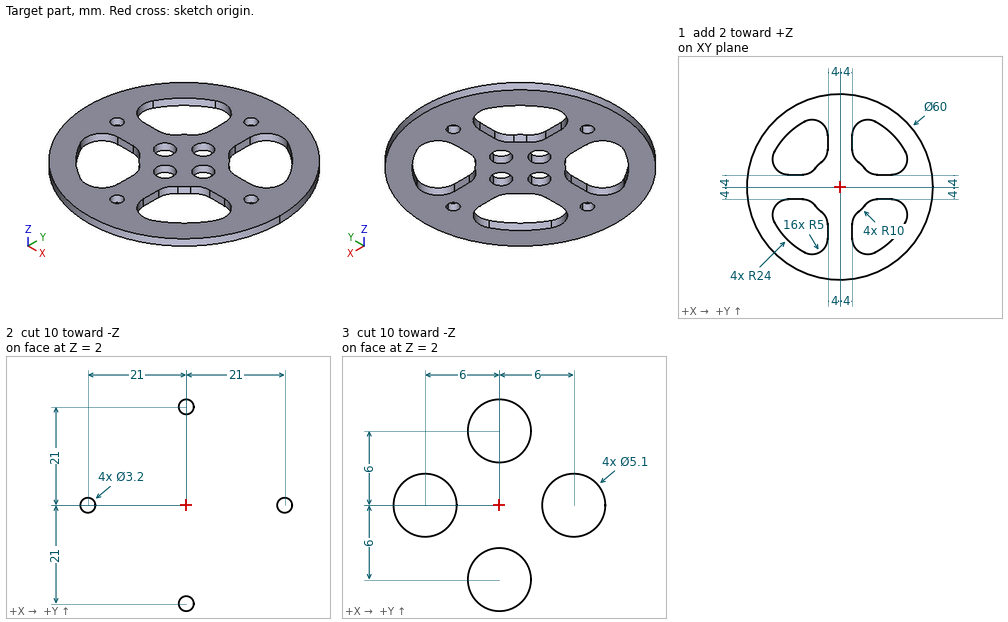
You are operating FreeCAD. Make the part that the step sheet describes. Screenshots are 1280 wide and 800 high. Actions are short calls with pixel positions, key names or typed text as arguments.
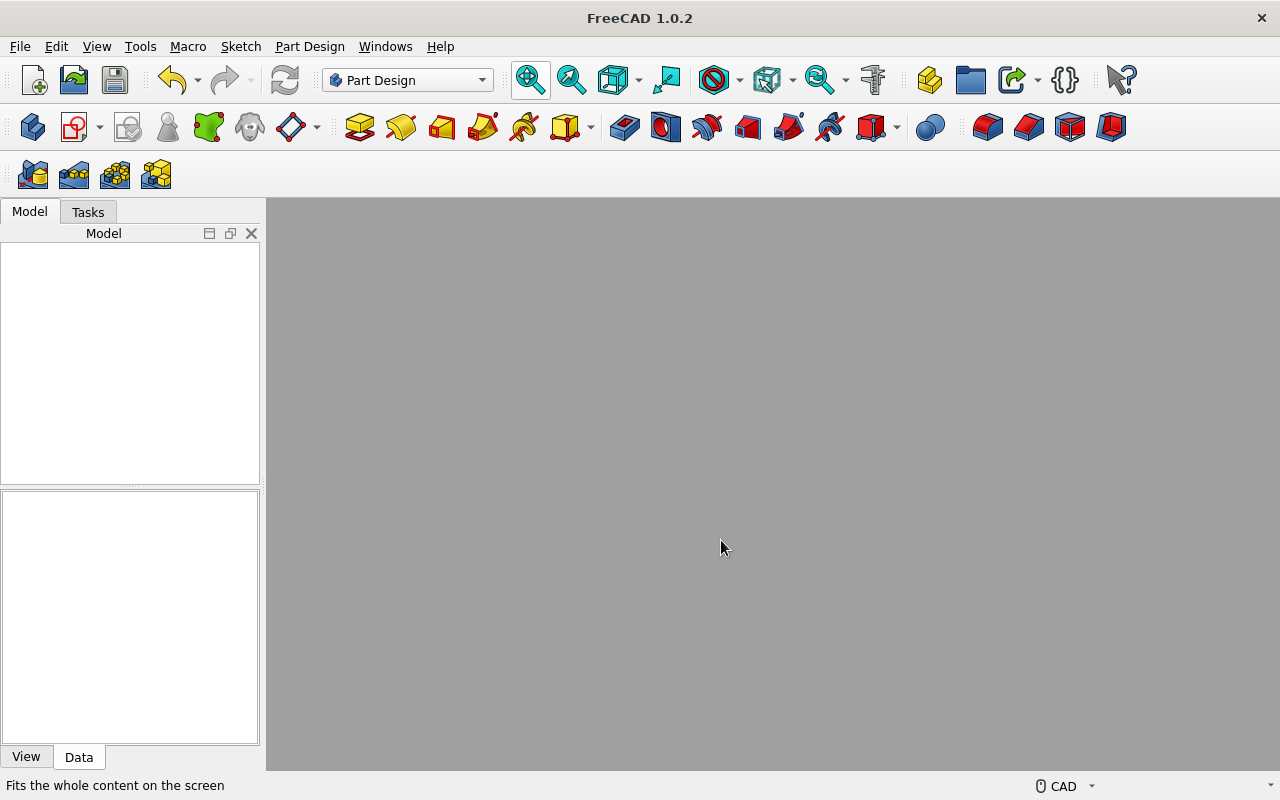
key(ctrl+n)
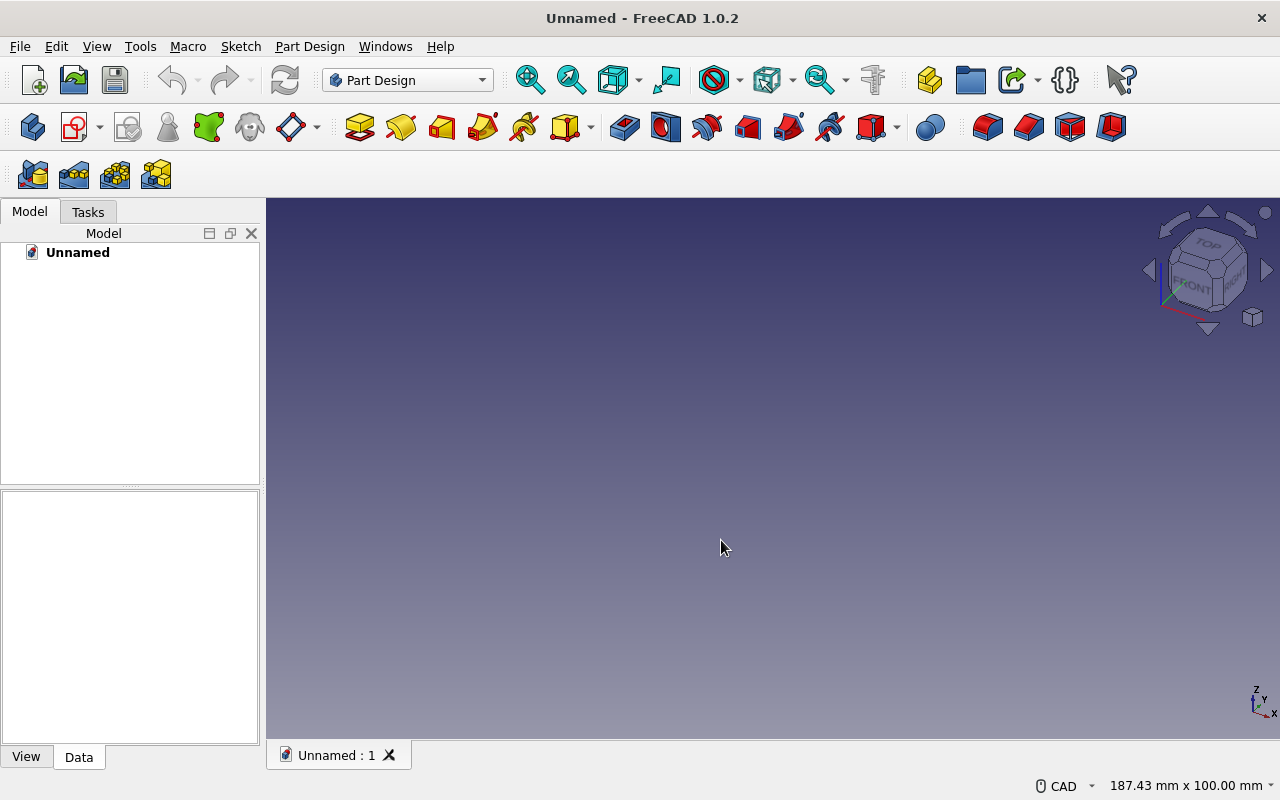
click(74, 128)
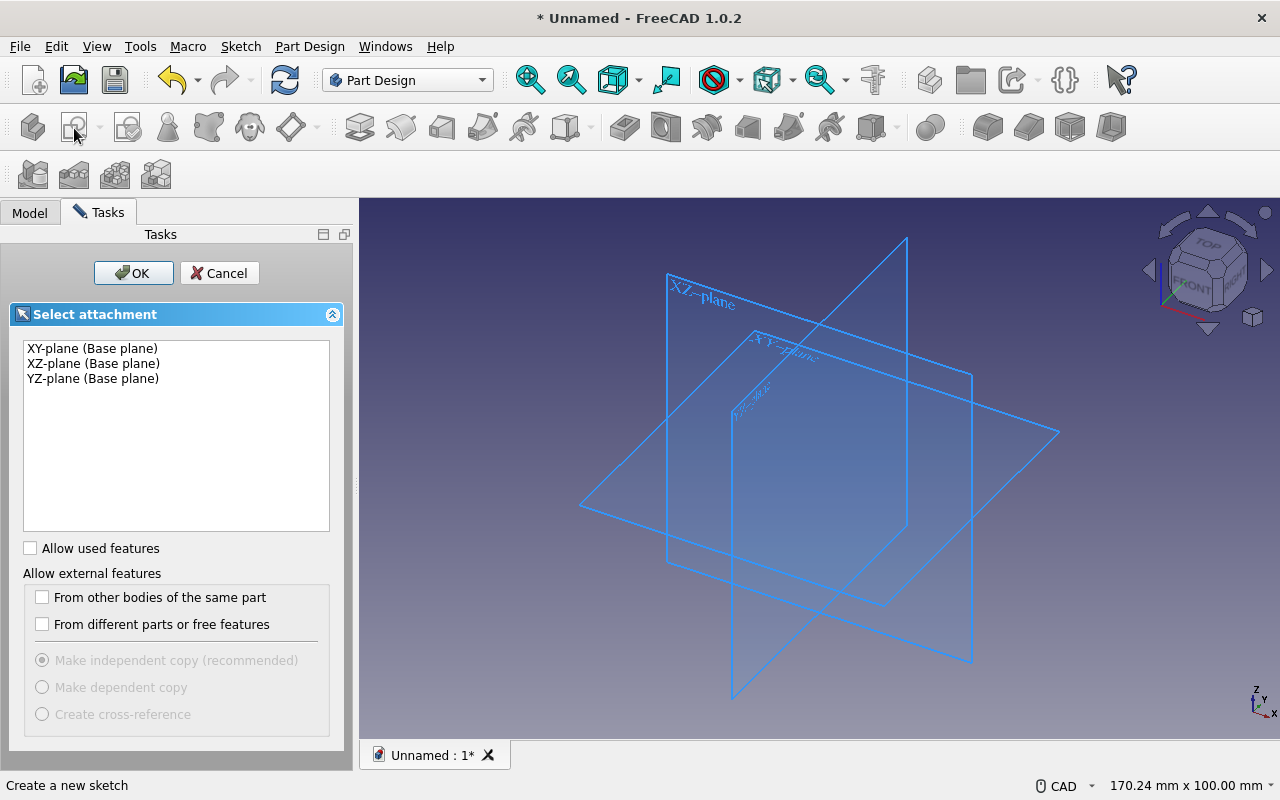
click(84, 348)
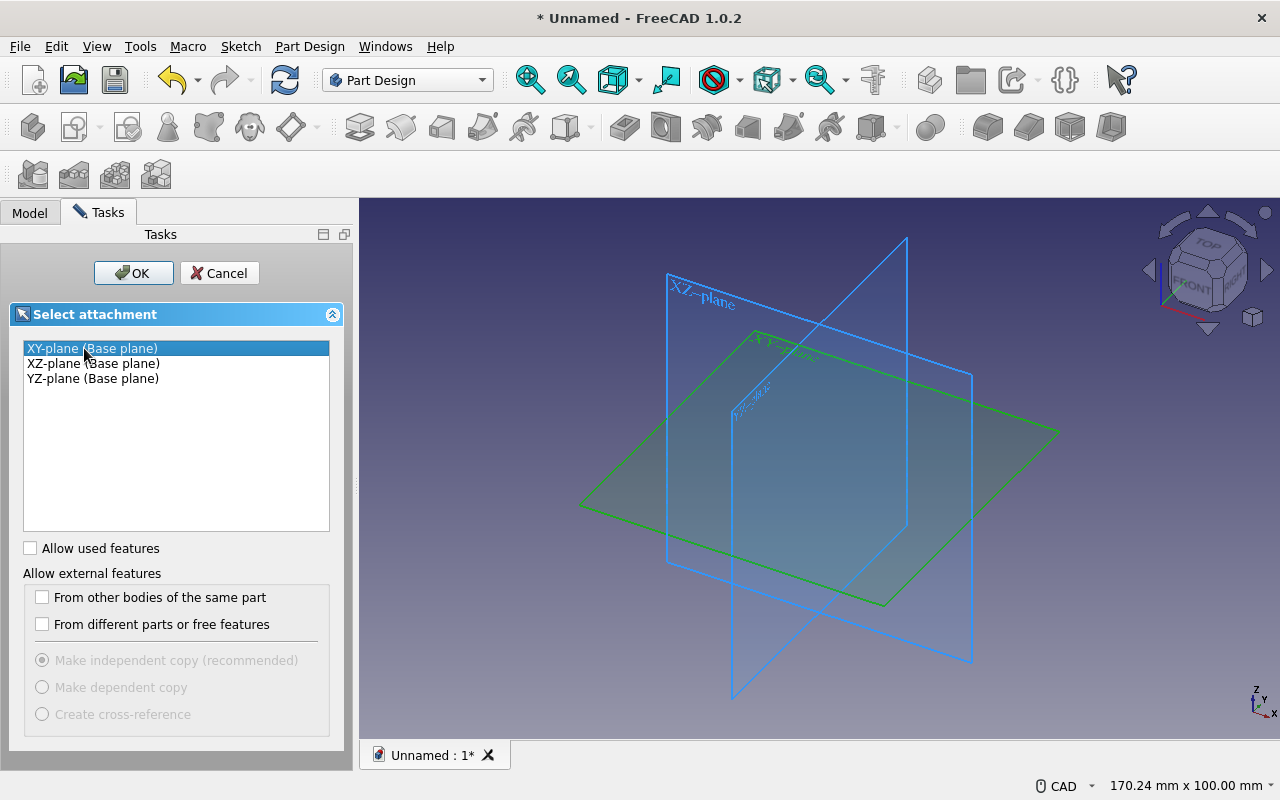
click(134, 273)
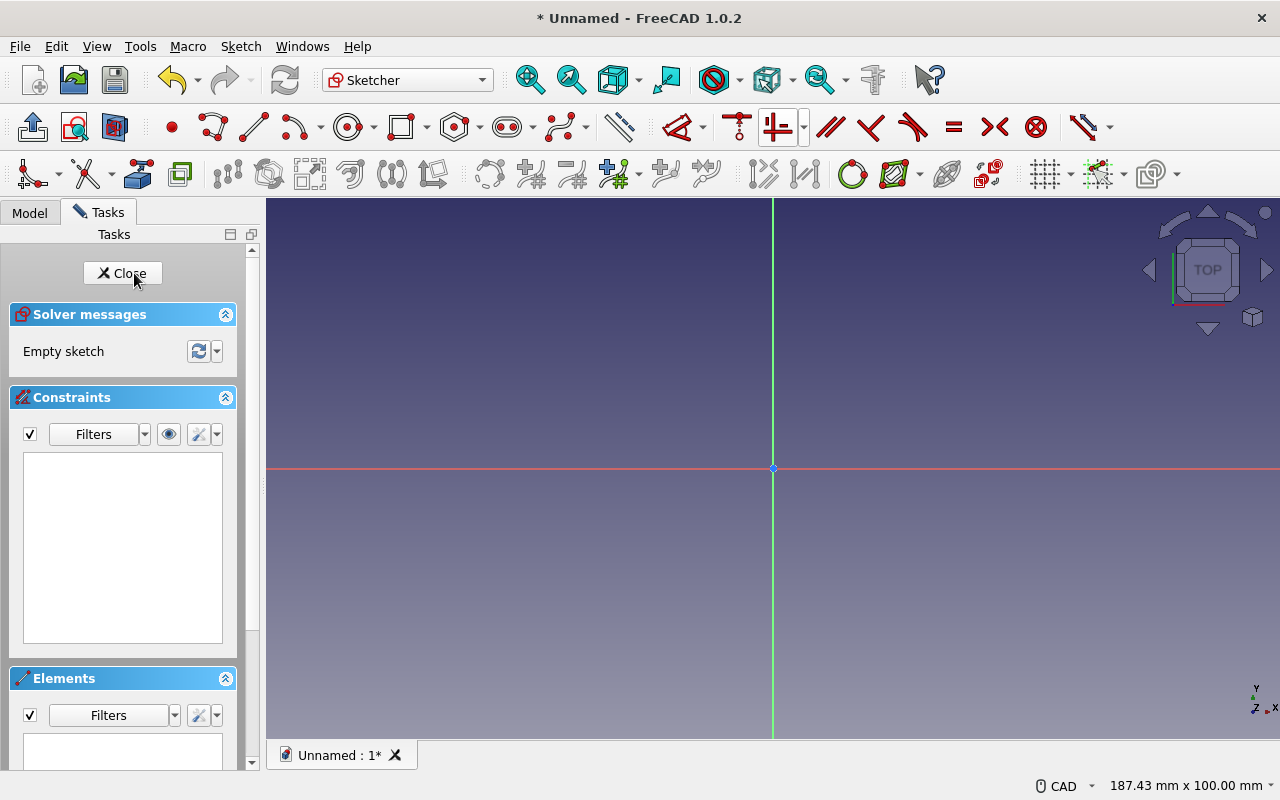
click(254, 128)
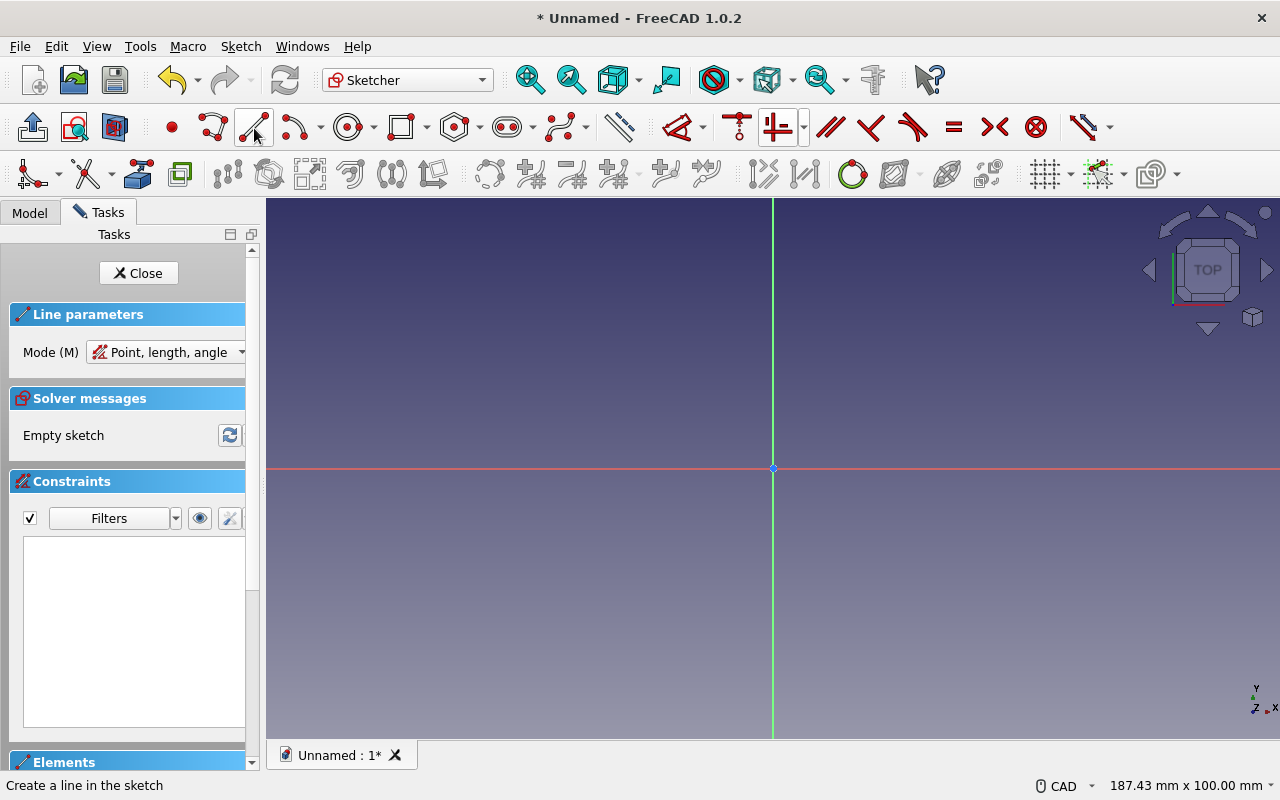
click(751, 533)
click(751, 559)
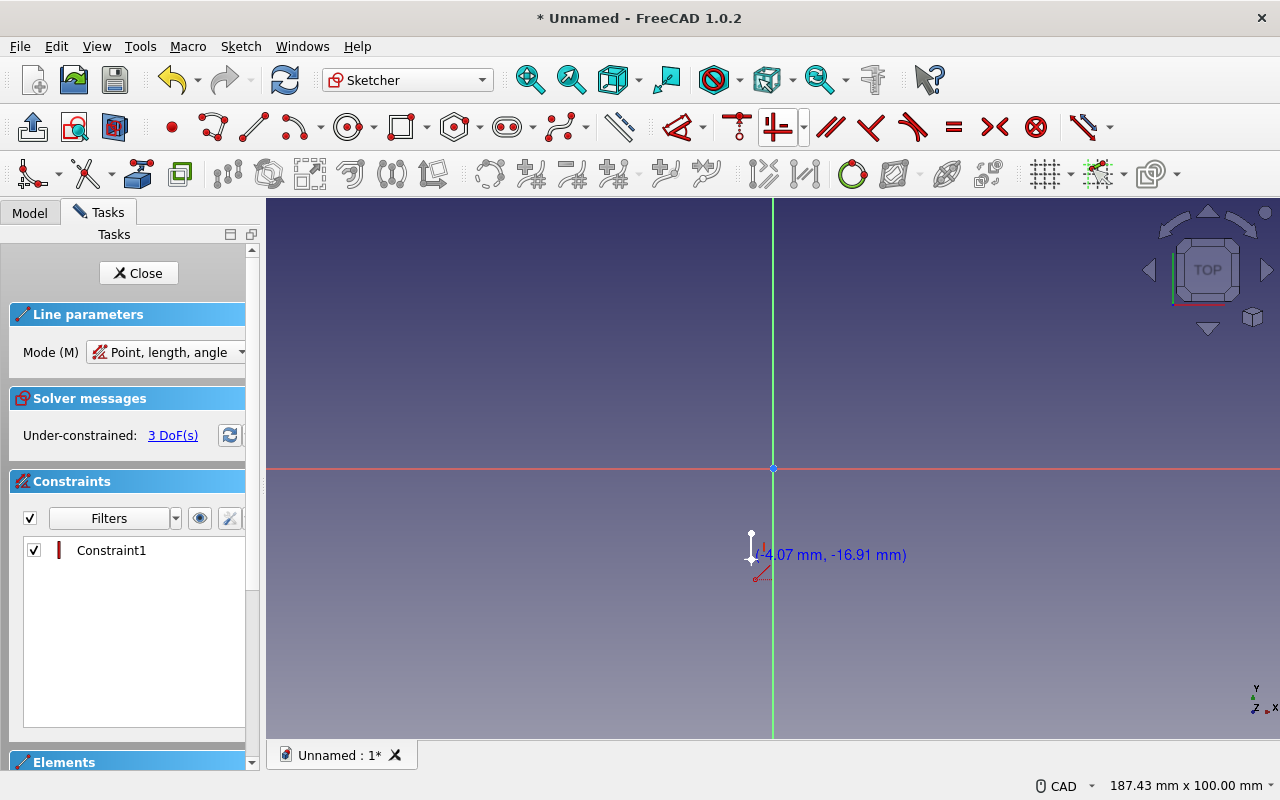
click(682, 490)
click(708, 490)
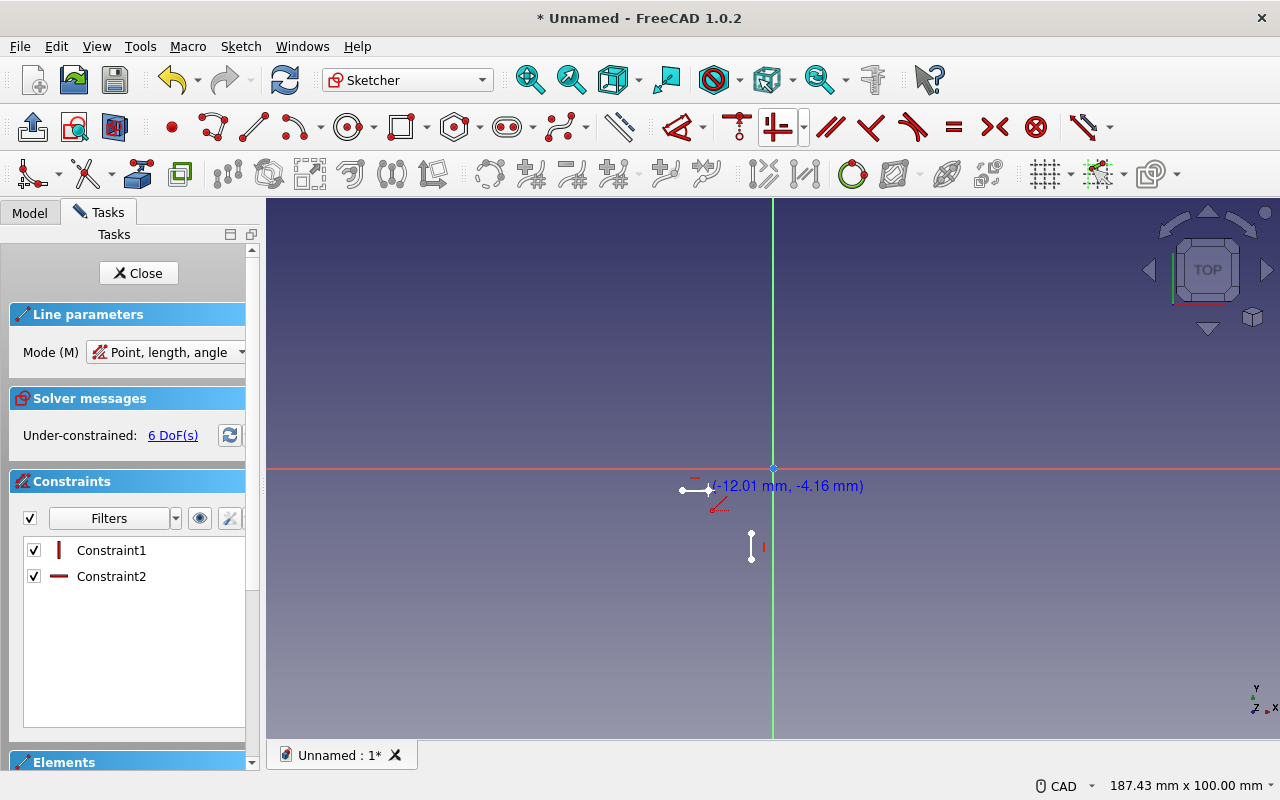
click(320, 128)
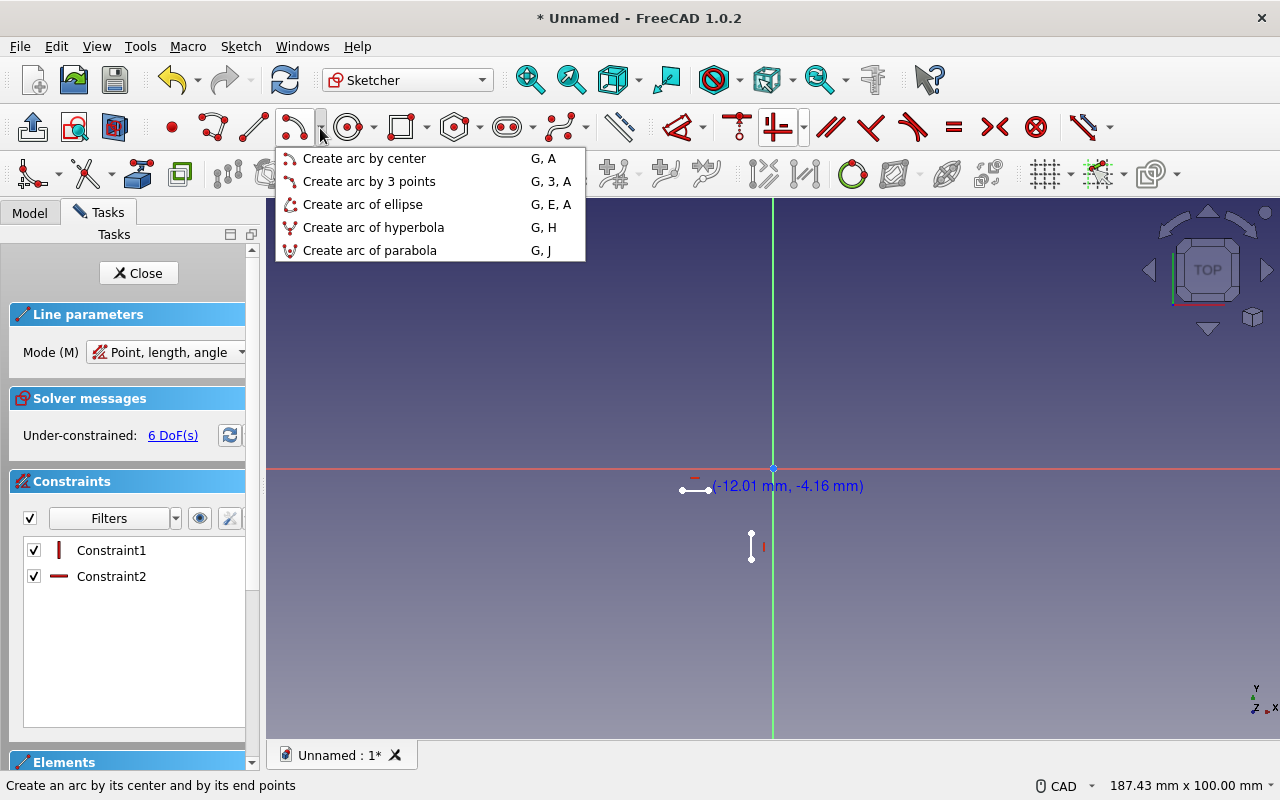
click(430, 182)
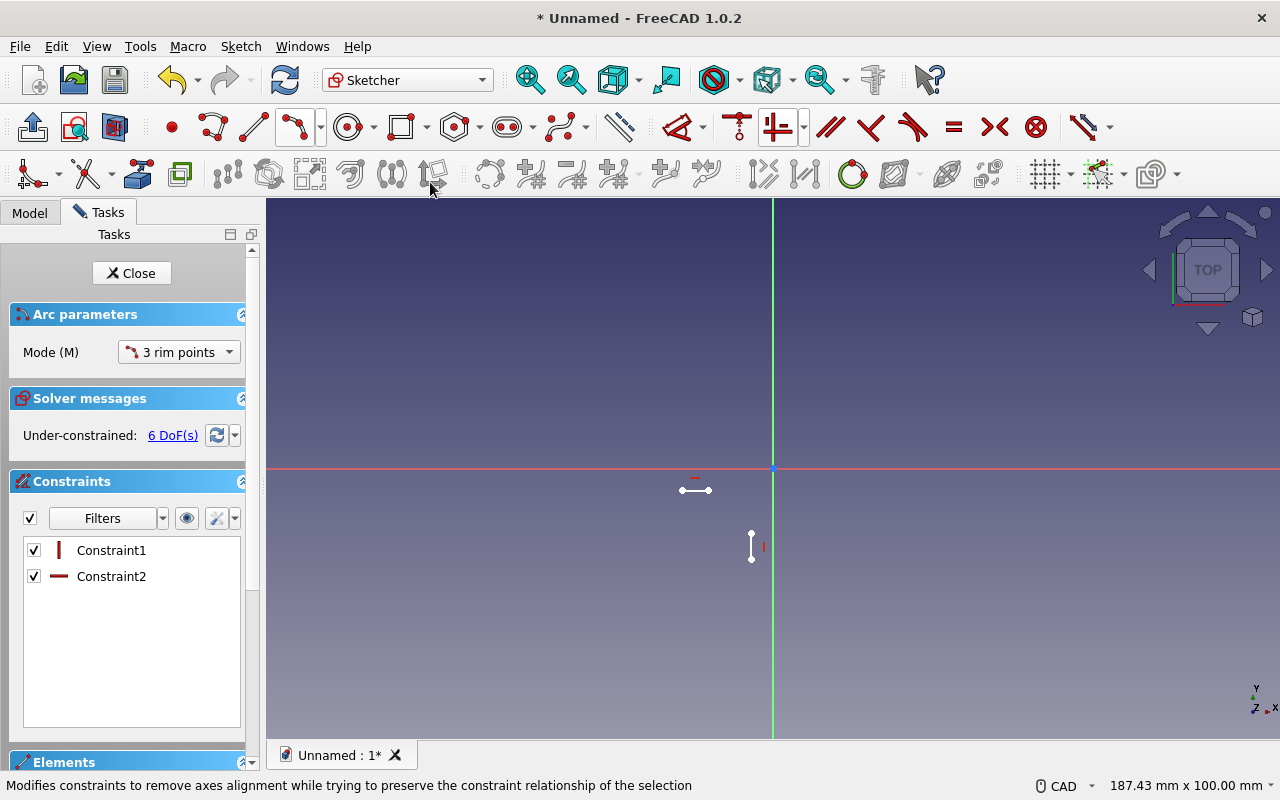
scroll(751, 559, up, 2)